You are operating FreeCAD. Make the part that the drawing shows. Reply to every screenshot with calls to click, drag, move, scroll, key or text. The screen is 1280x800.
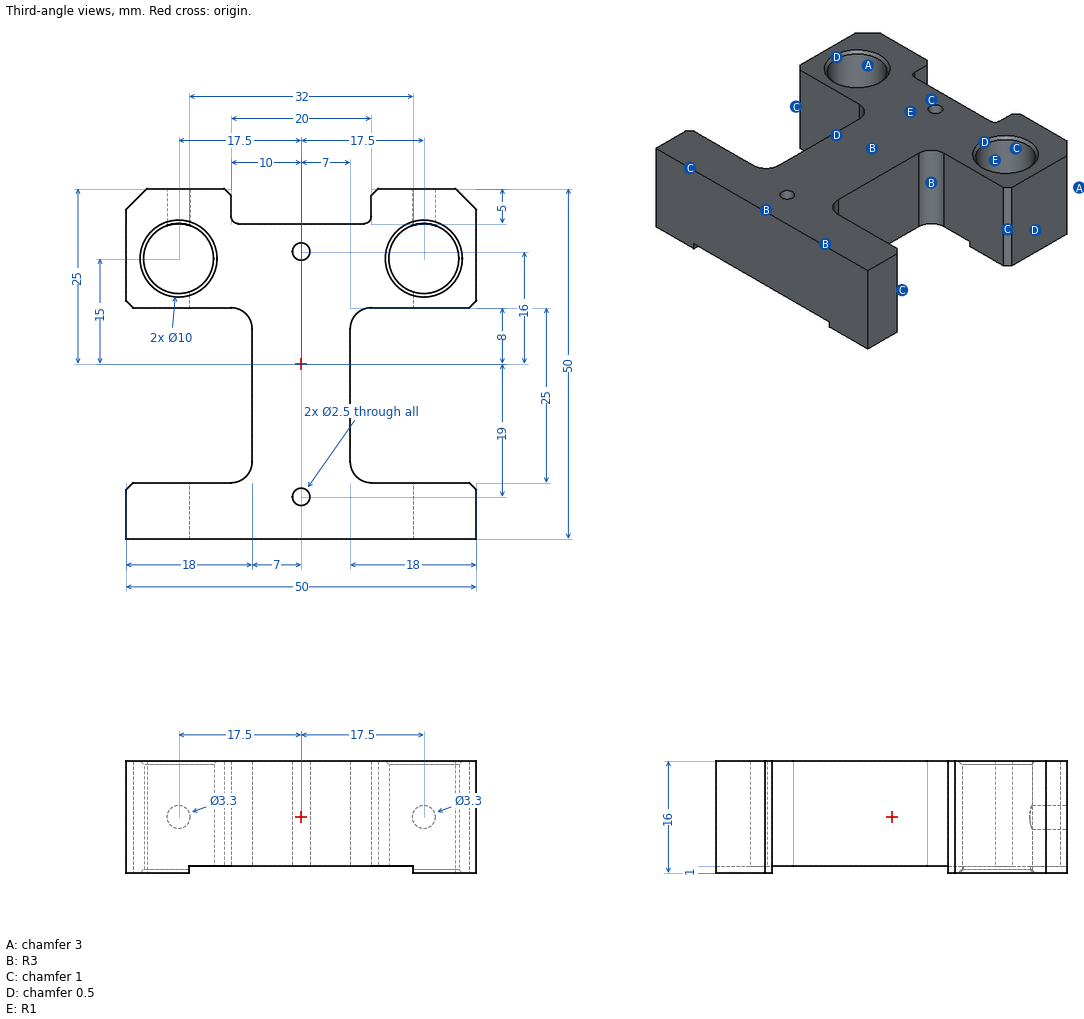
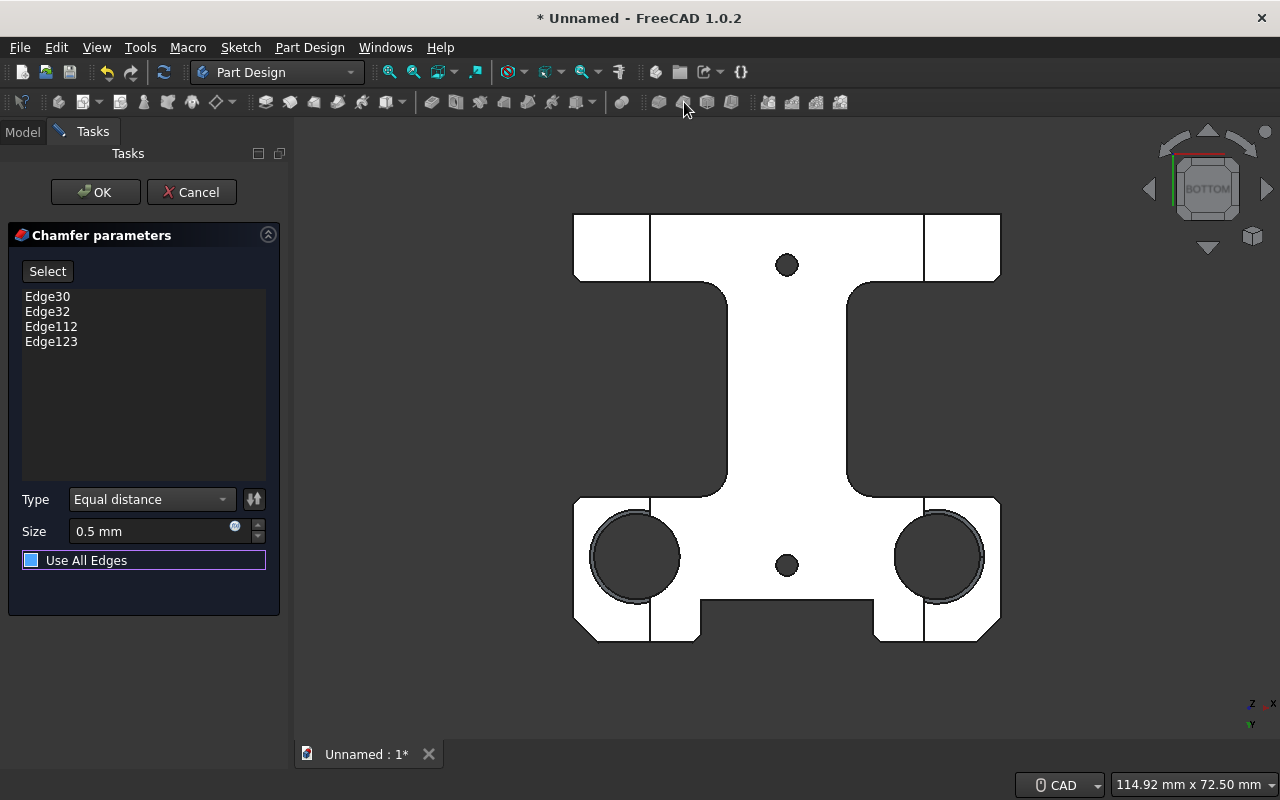
click(96, 192)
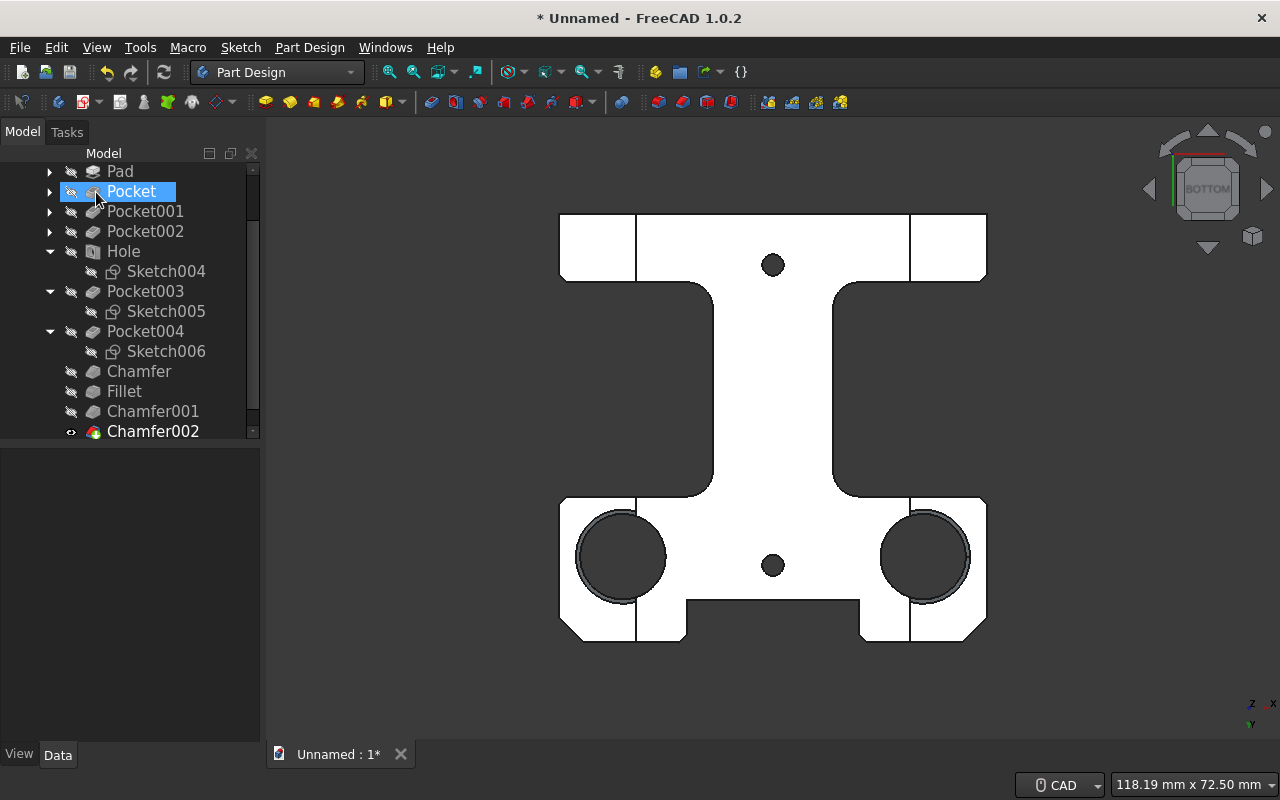
key(0)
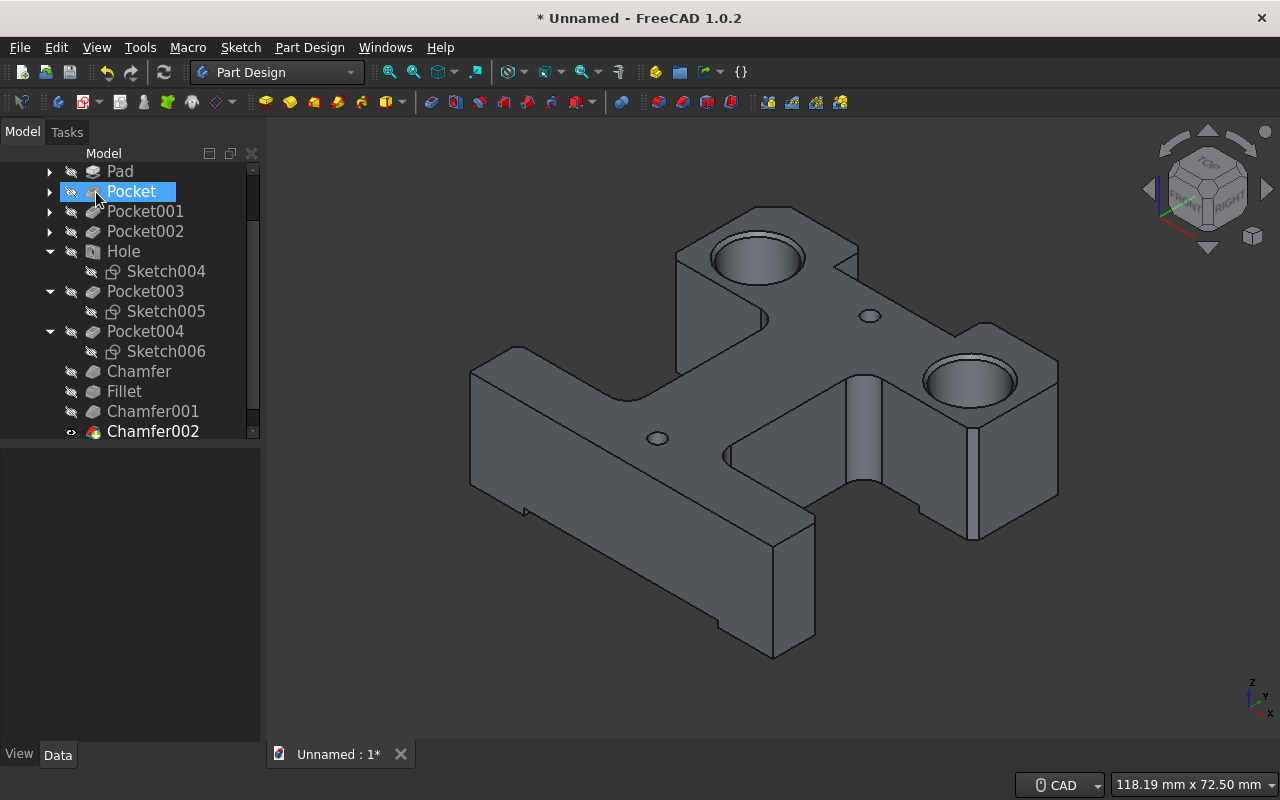
key(2)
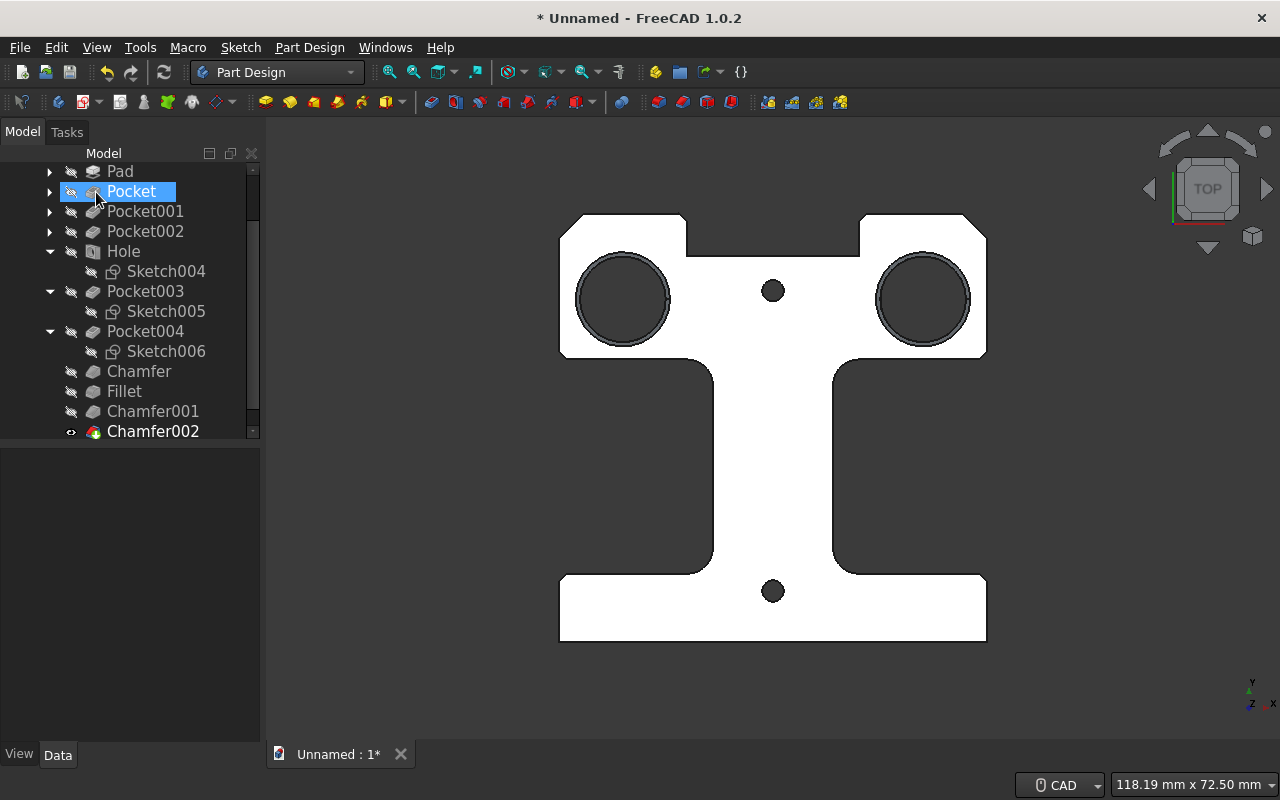
key(1)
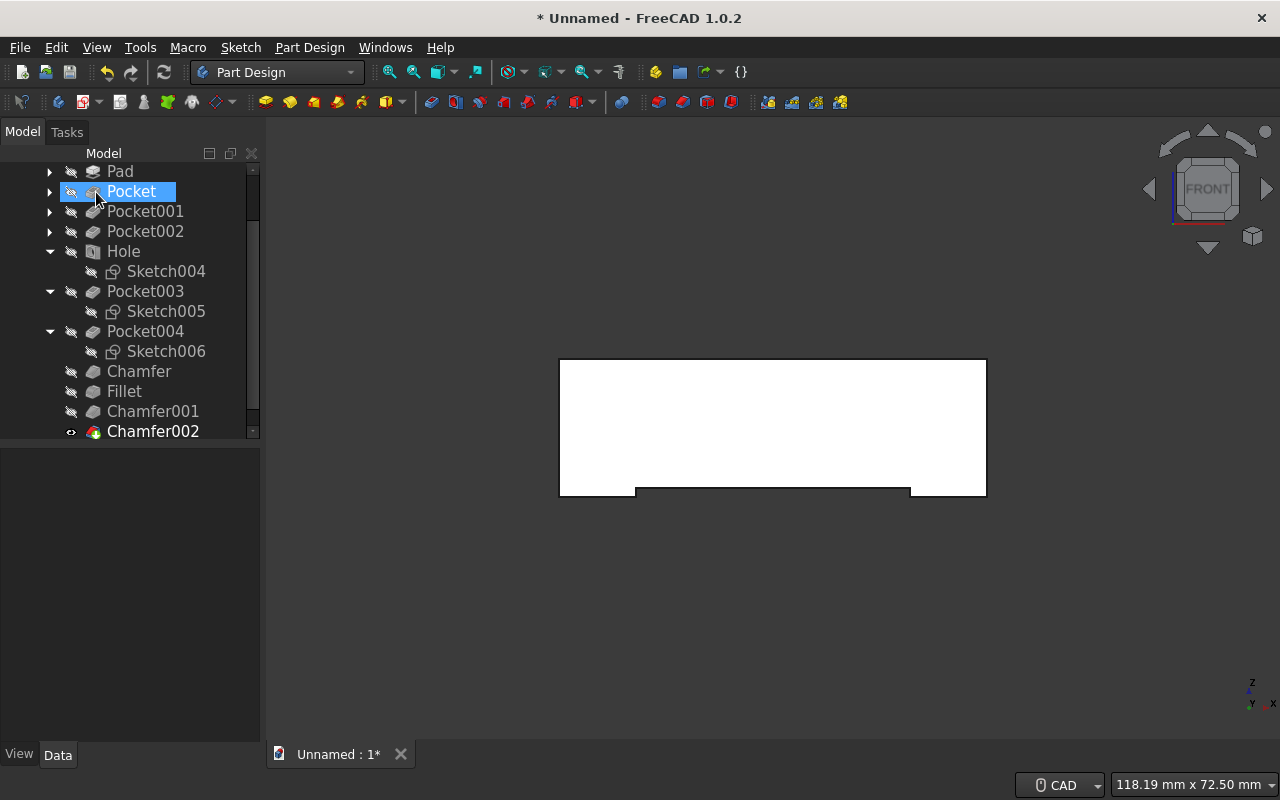
click(390, 72)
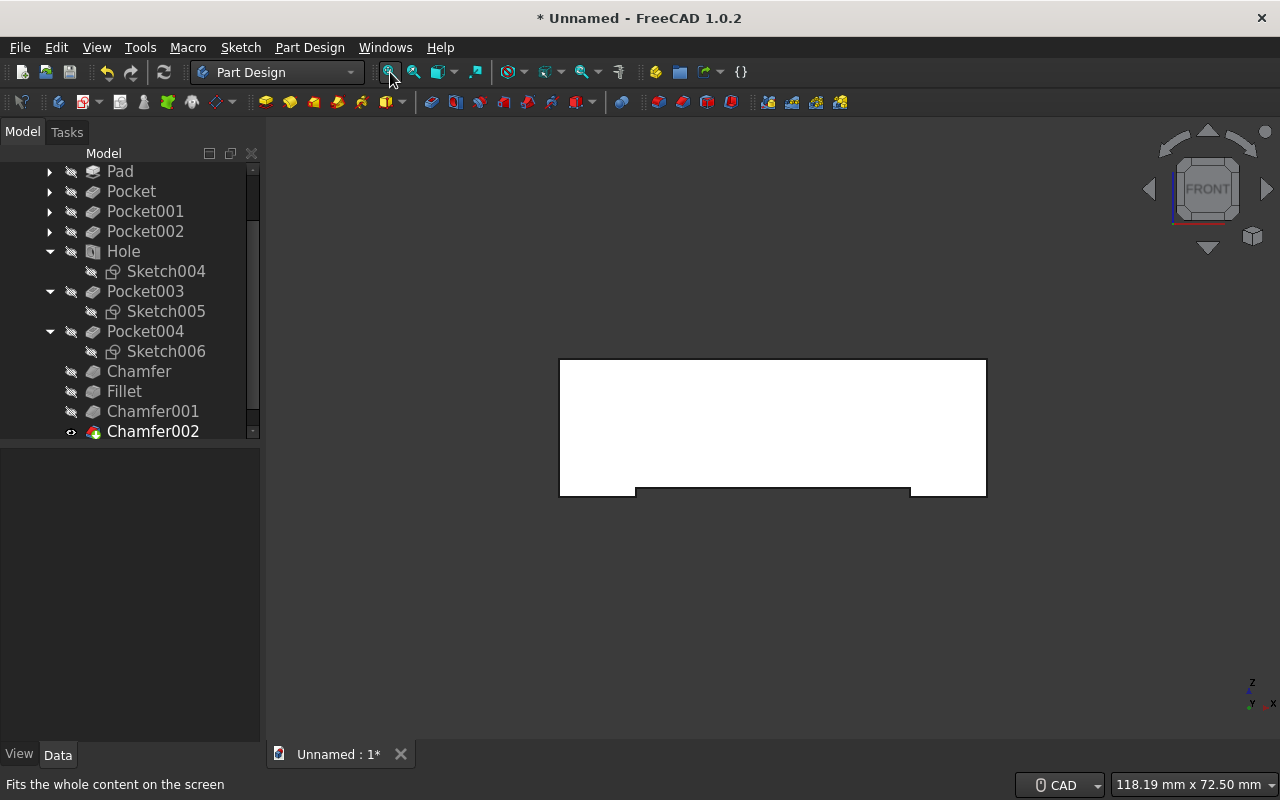
key(3)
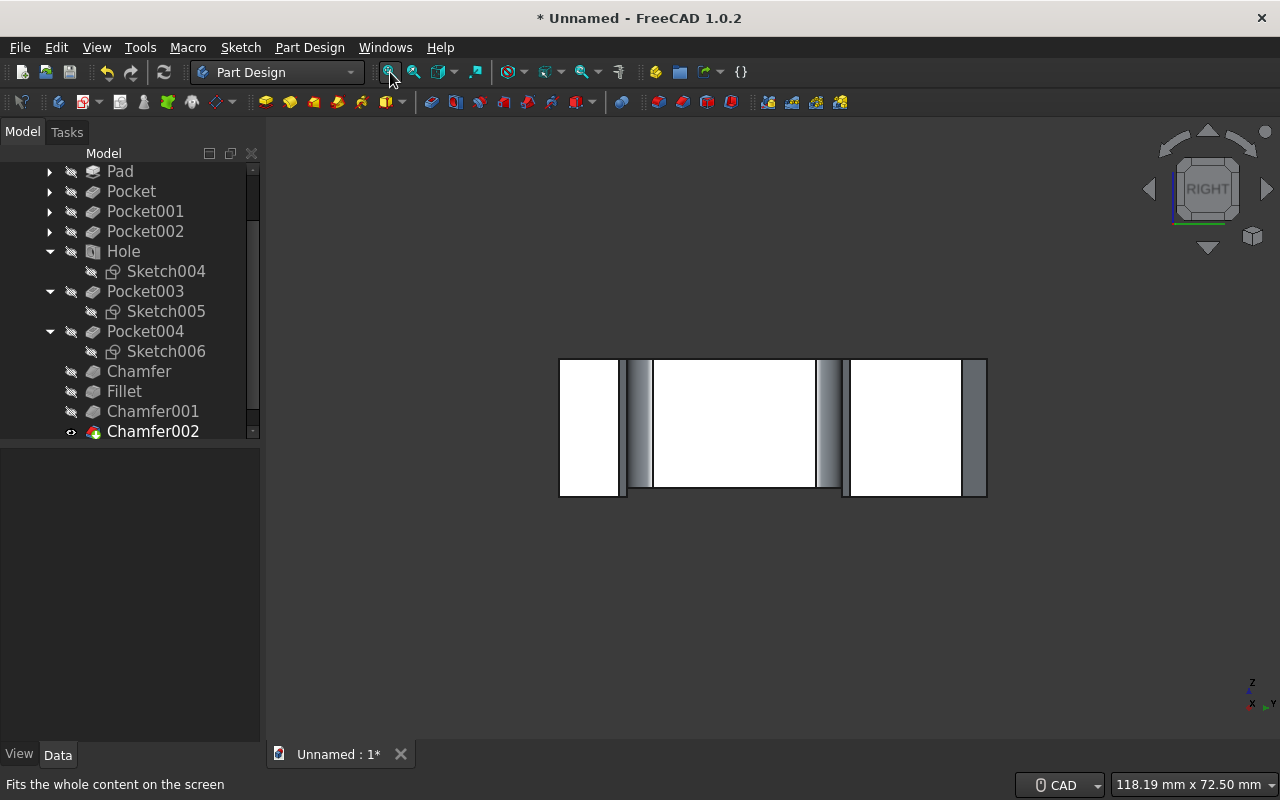
click(390, 72)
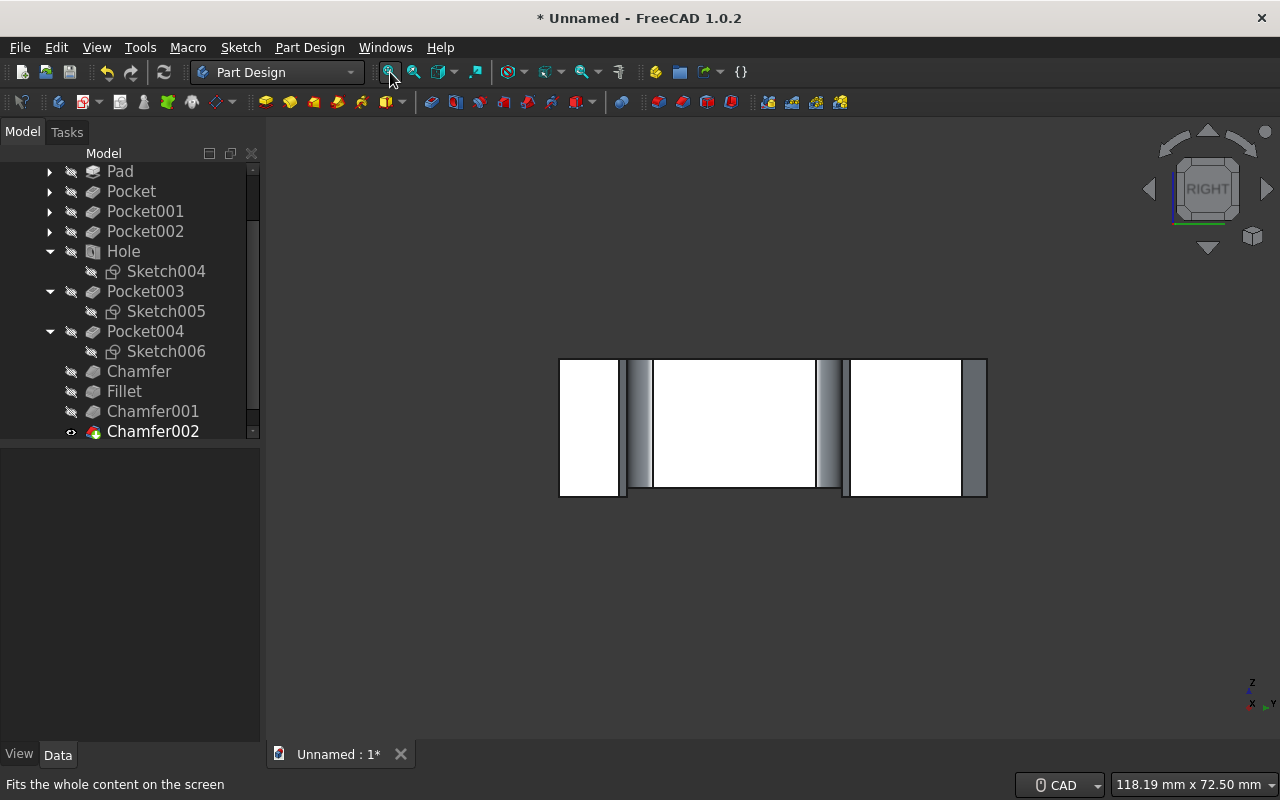
key(5)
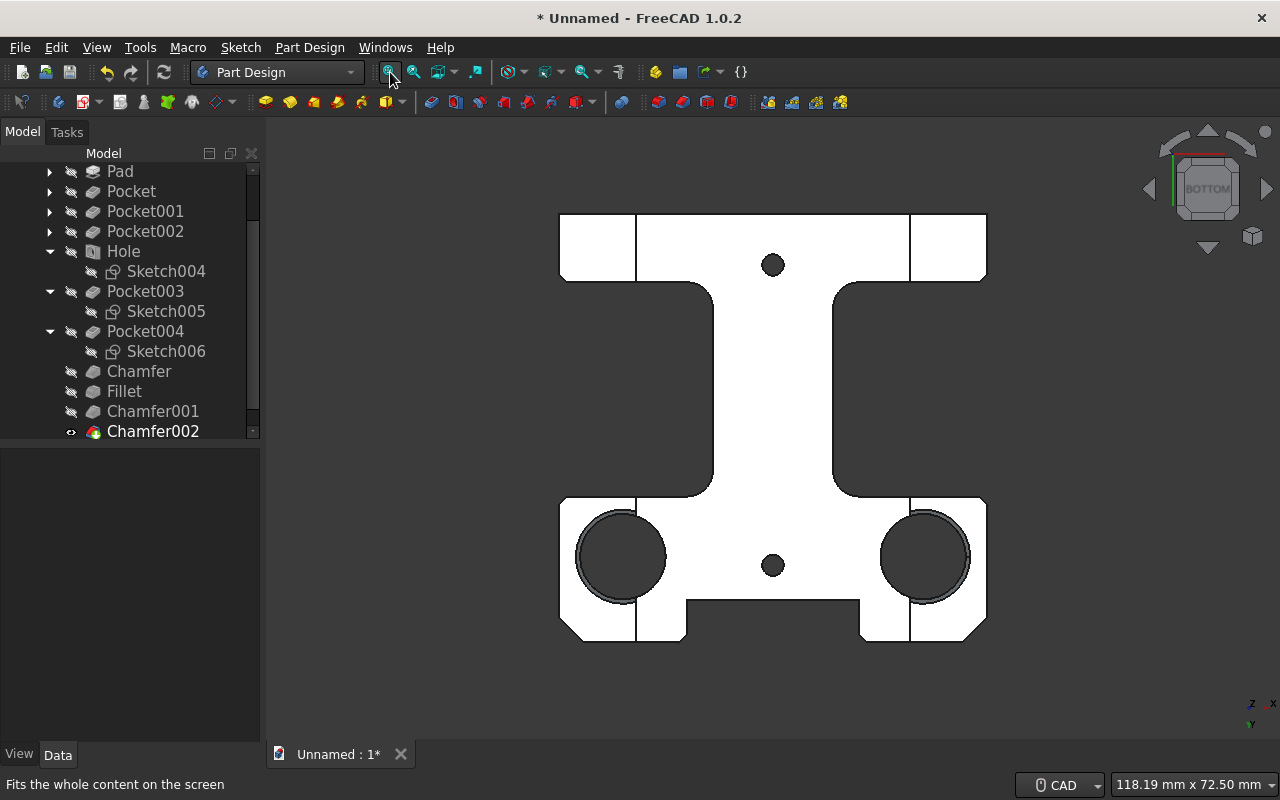
key(4)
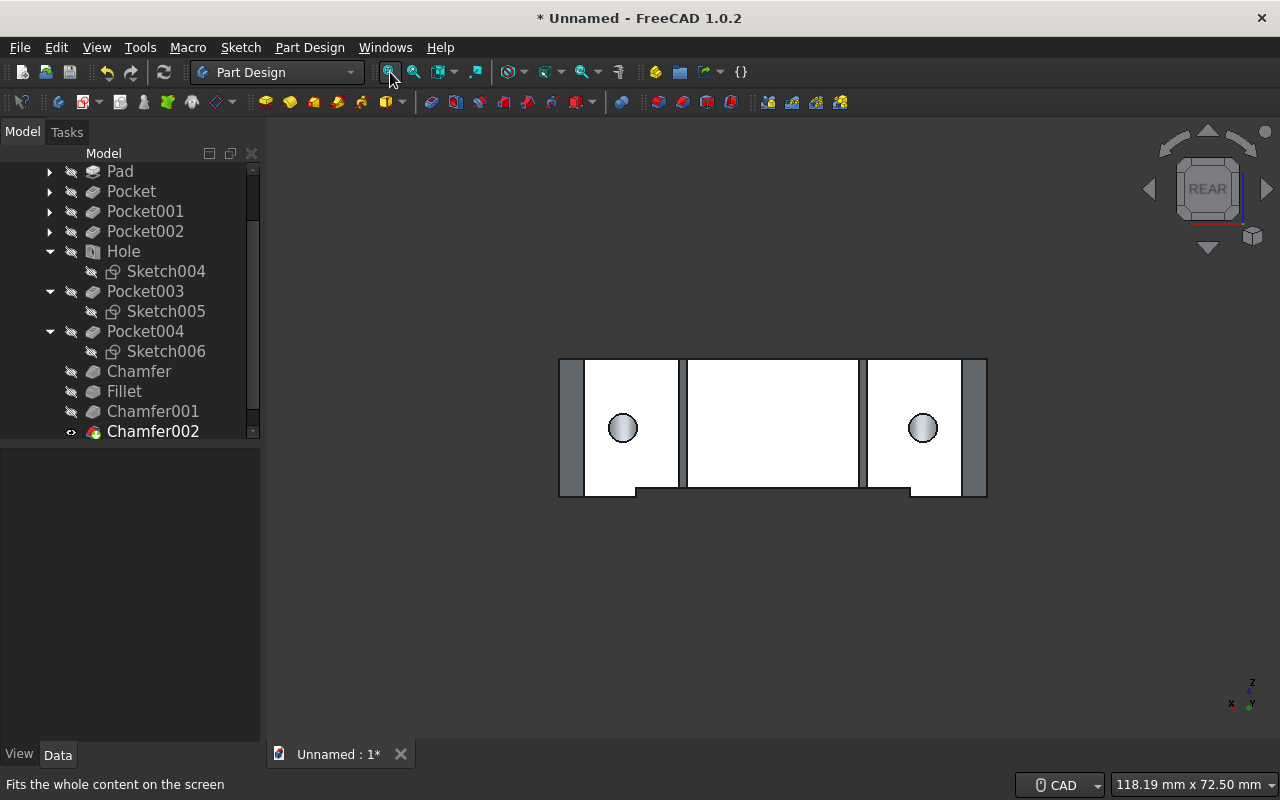
key(v)
key(f)